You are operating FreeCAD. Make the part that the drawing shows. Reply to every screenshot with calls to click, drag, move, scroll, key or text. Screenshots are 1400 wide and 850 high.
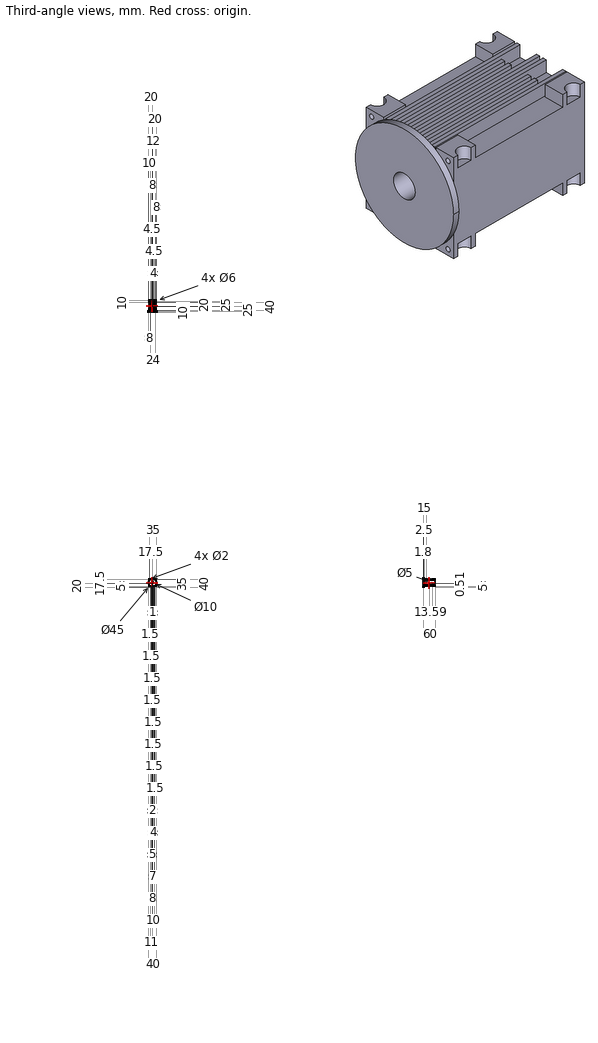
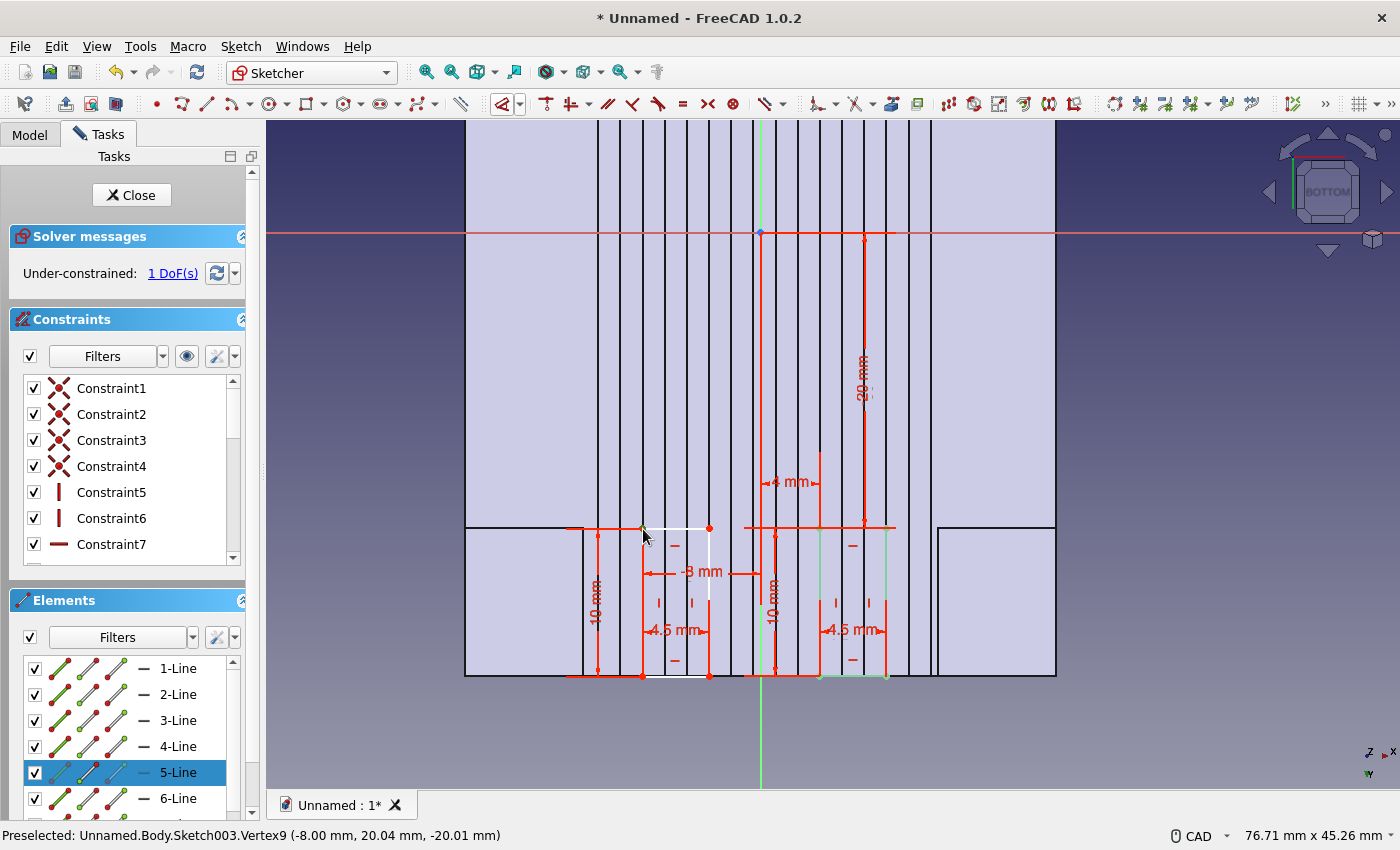
click(520, 104)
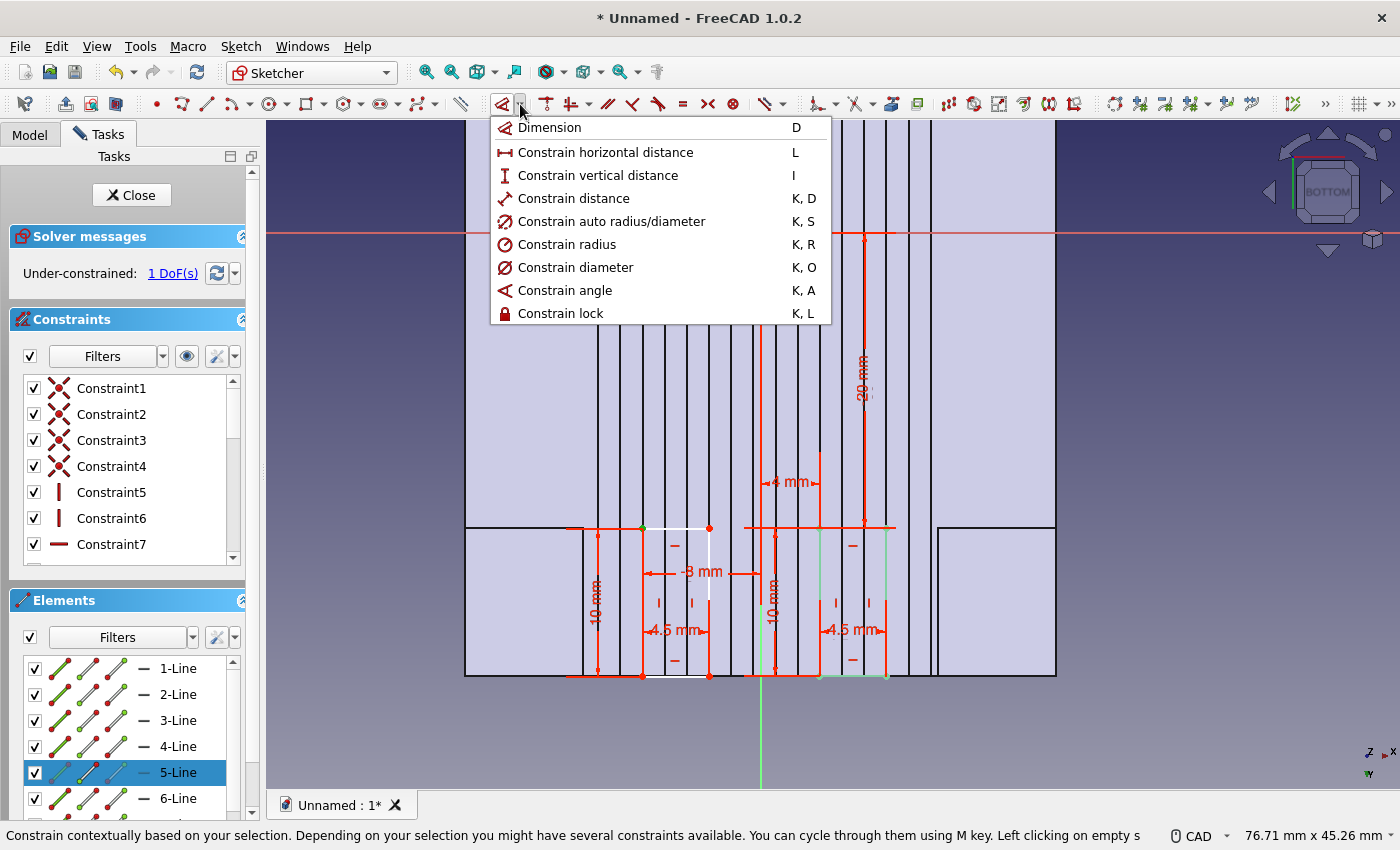
click(661, 176)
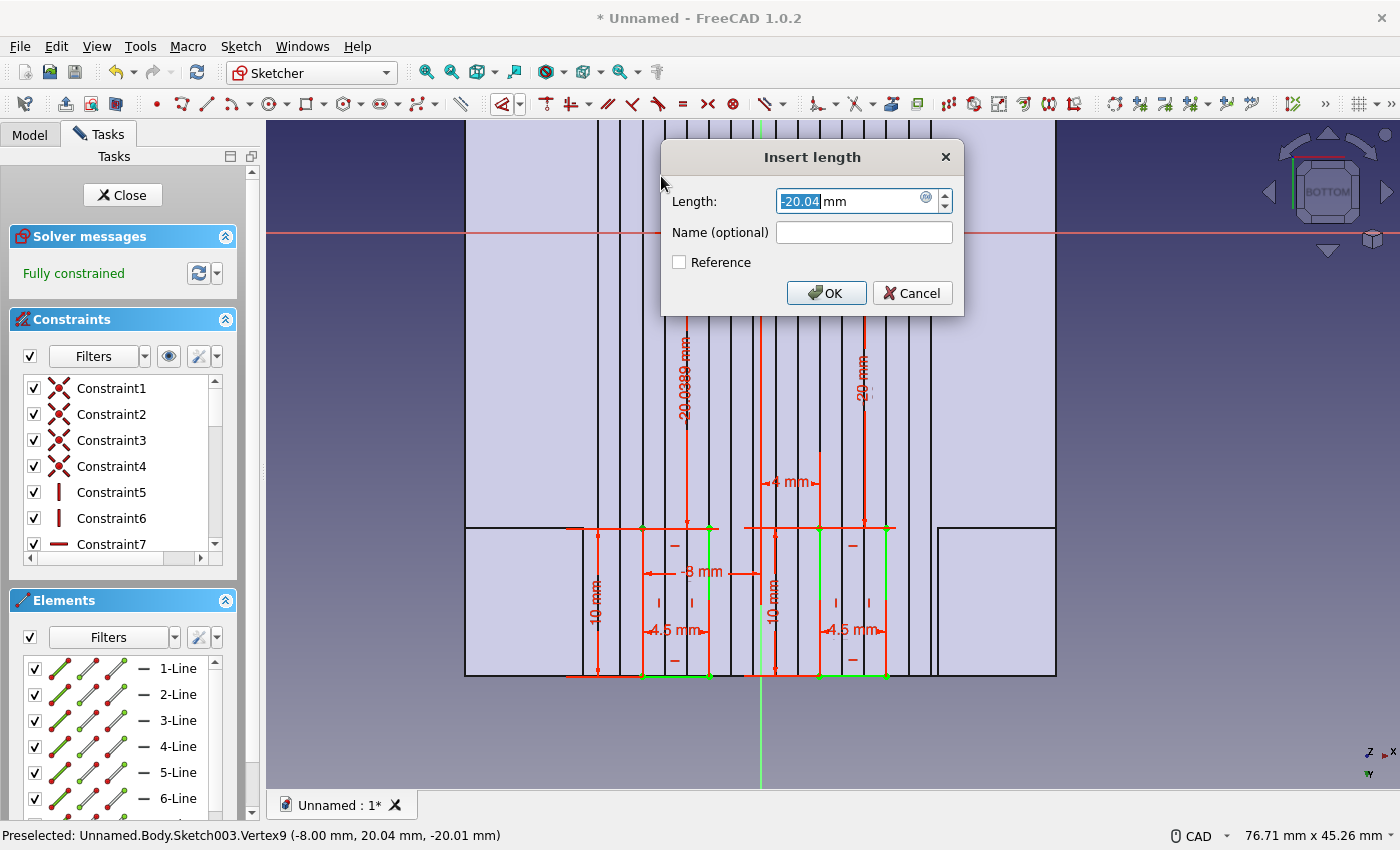
text(-20)
key(Return)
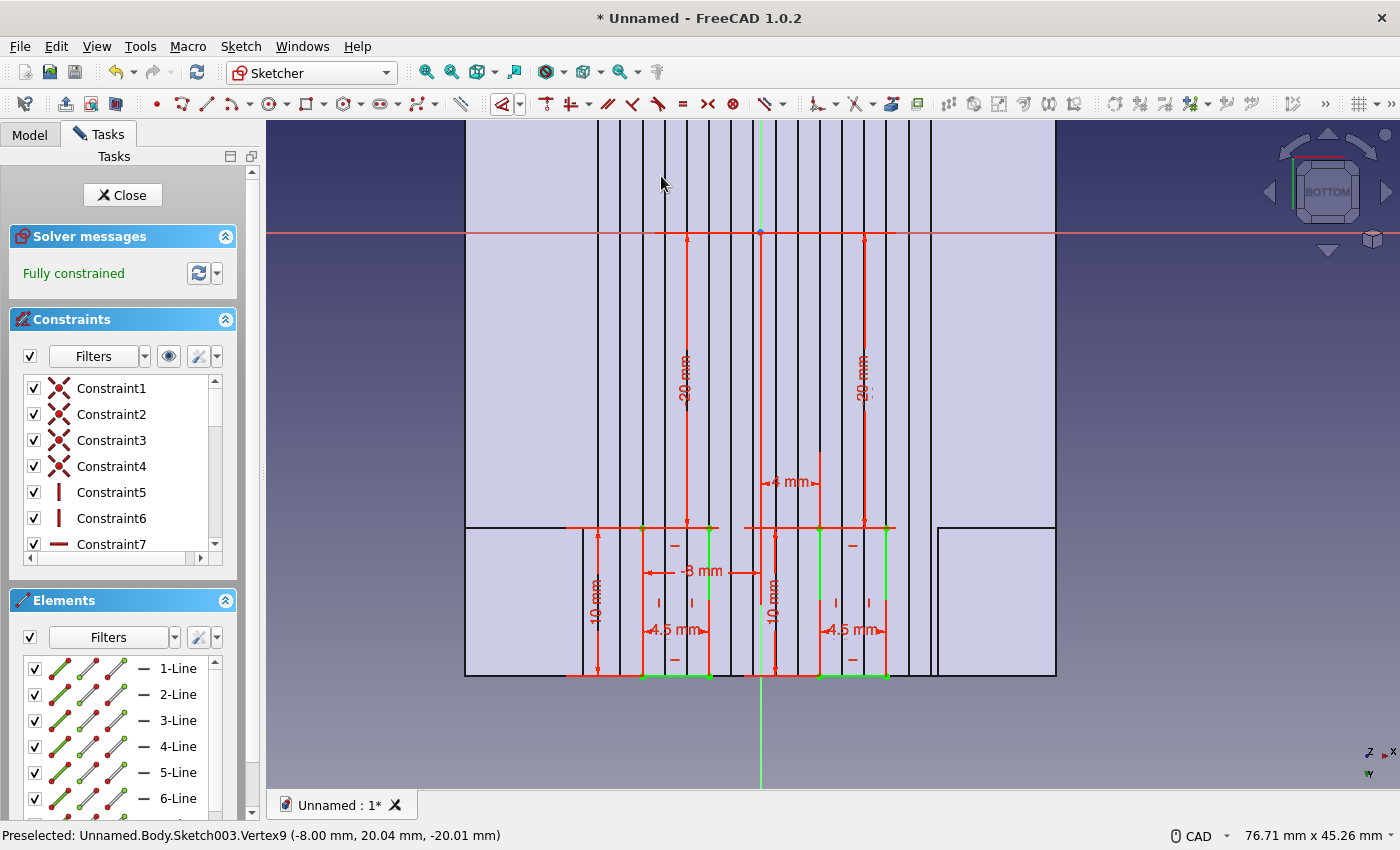
click(123, 195)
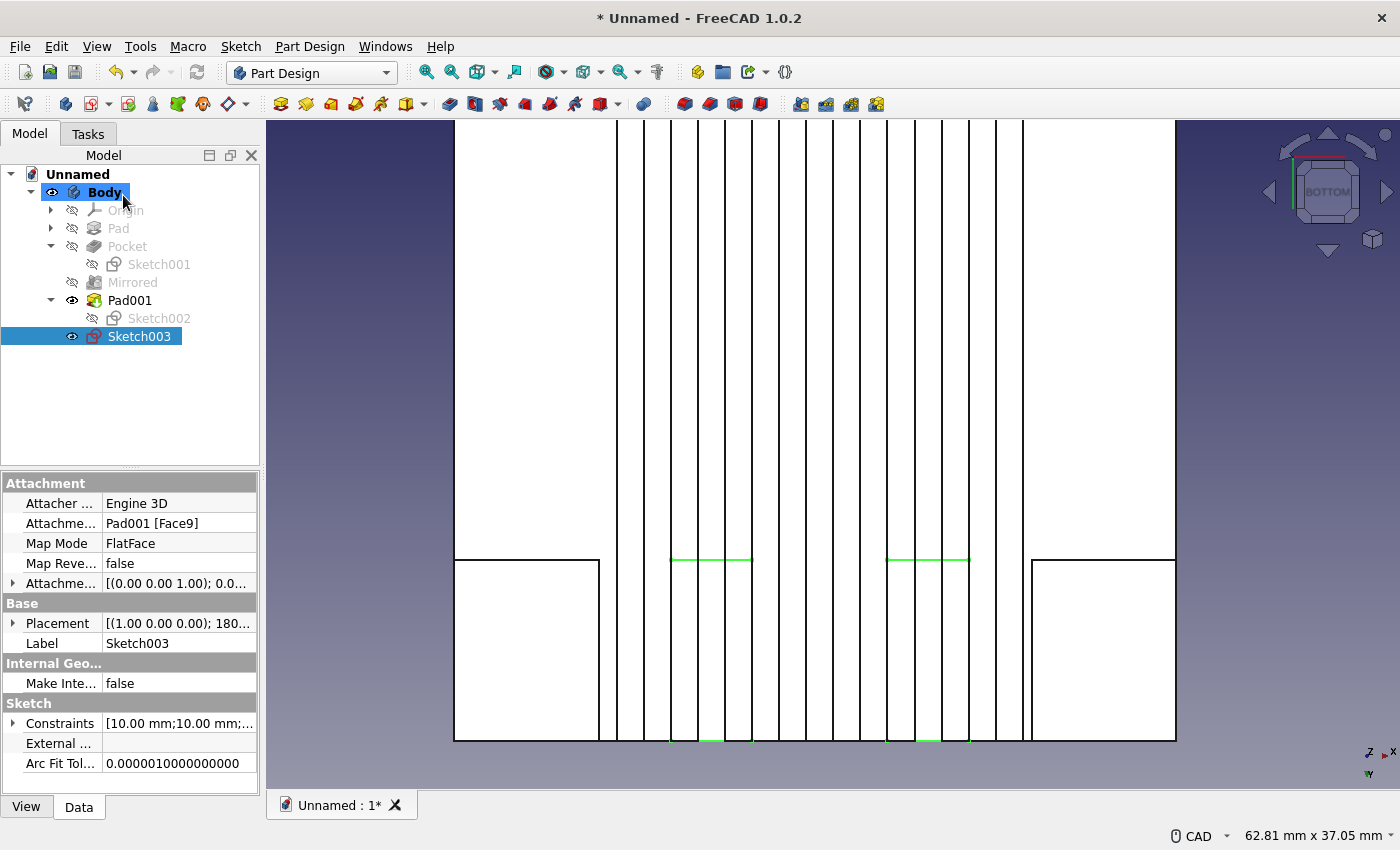
click(450, 104)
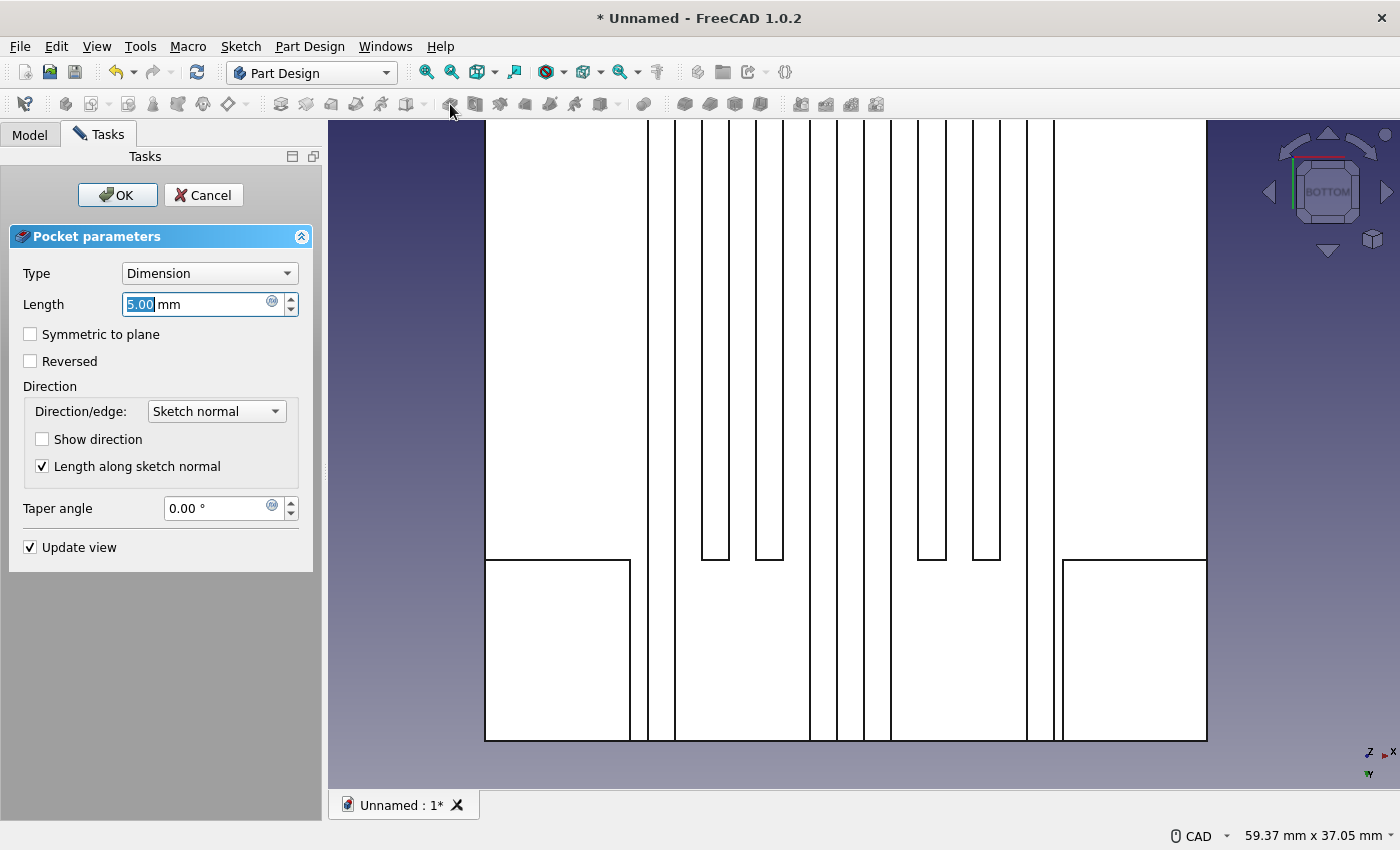
text(5)
key(Tab)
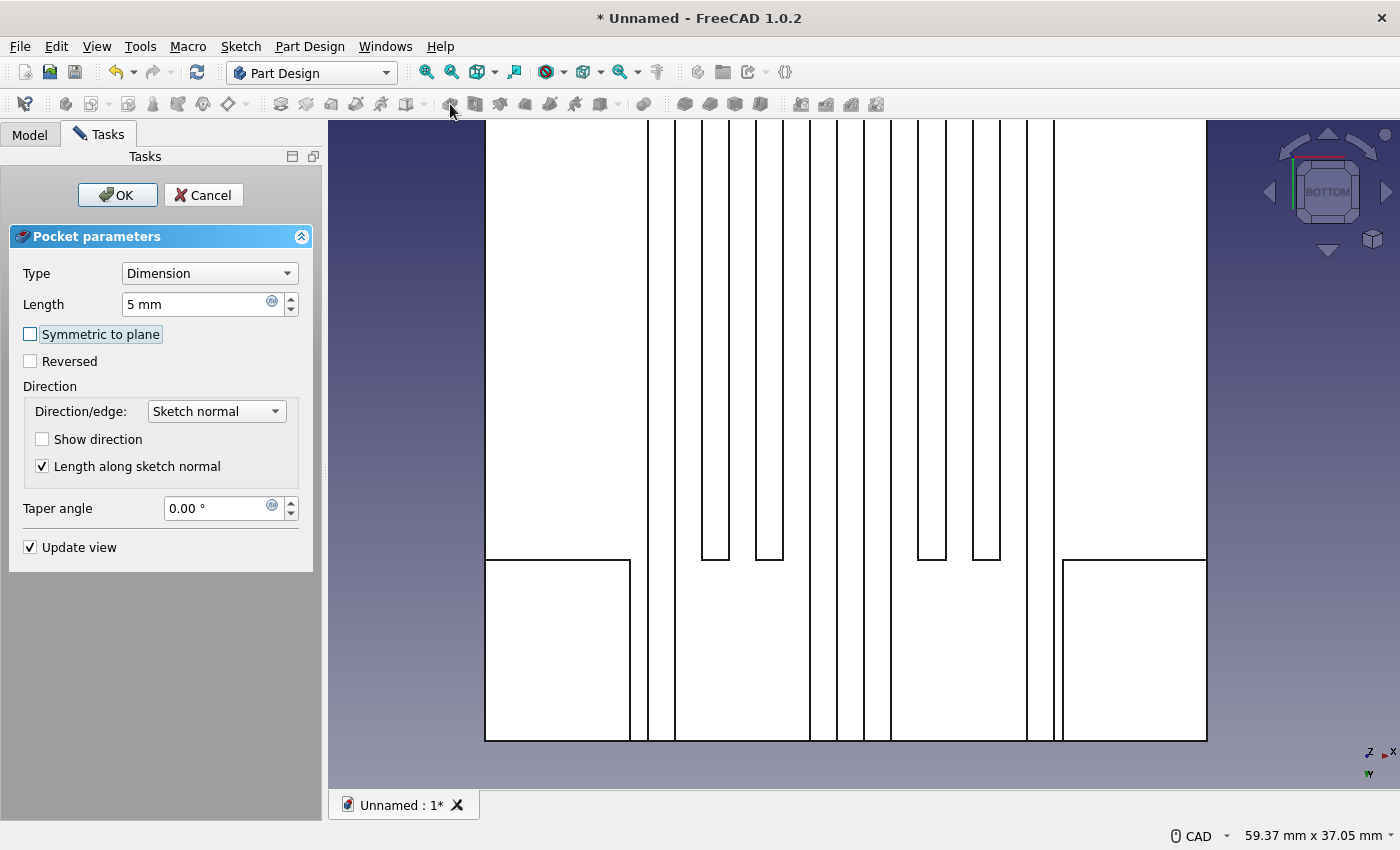
click(118, 195)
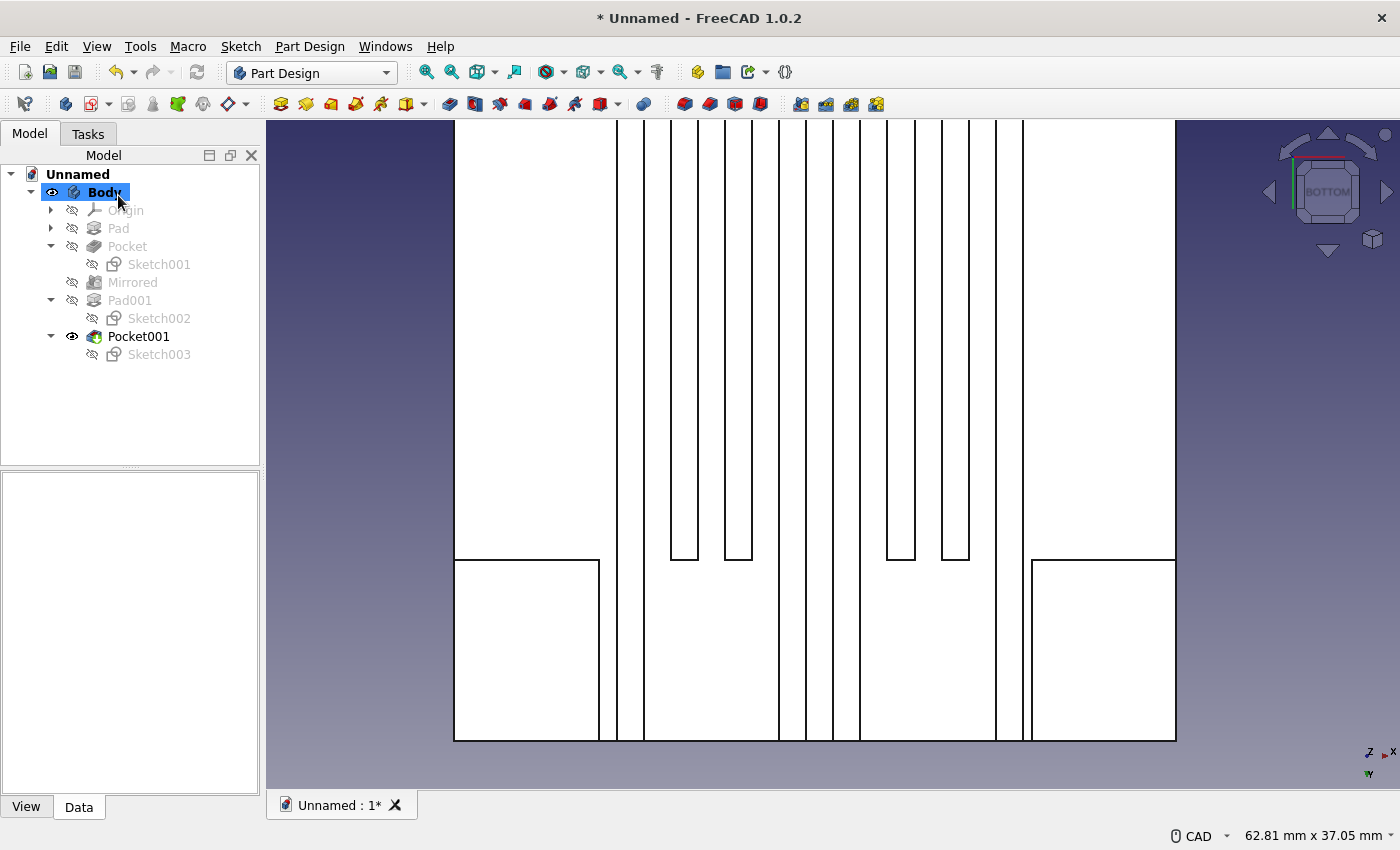
click(427, 72)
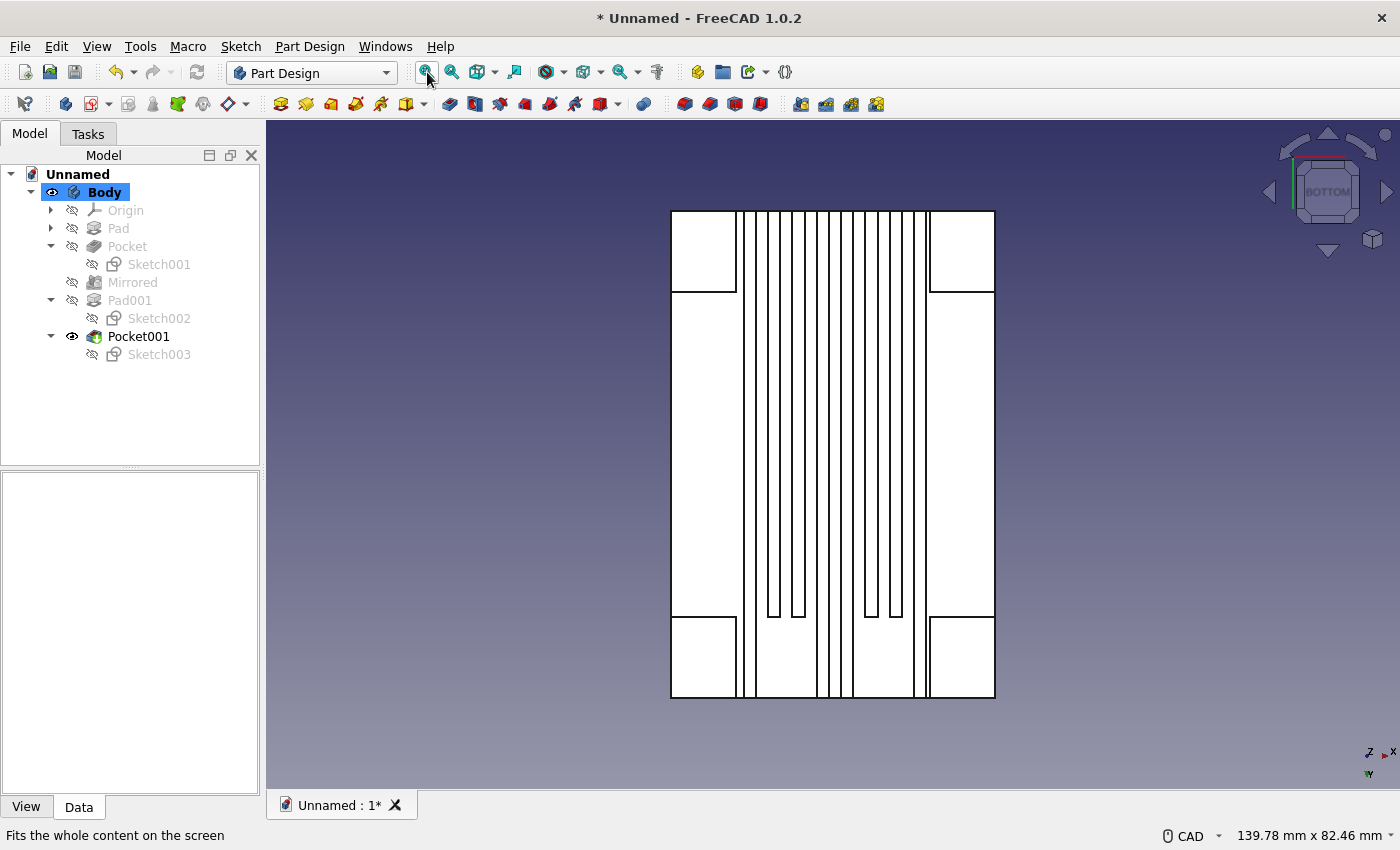
click(117, 300)